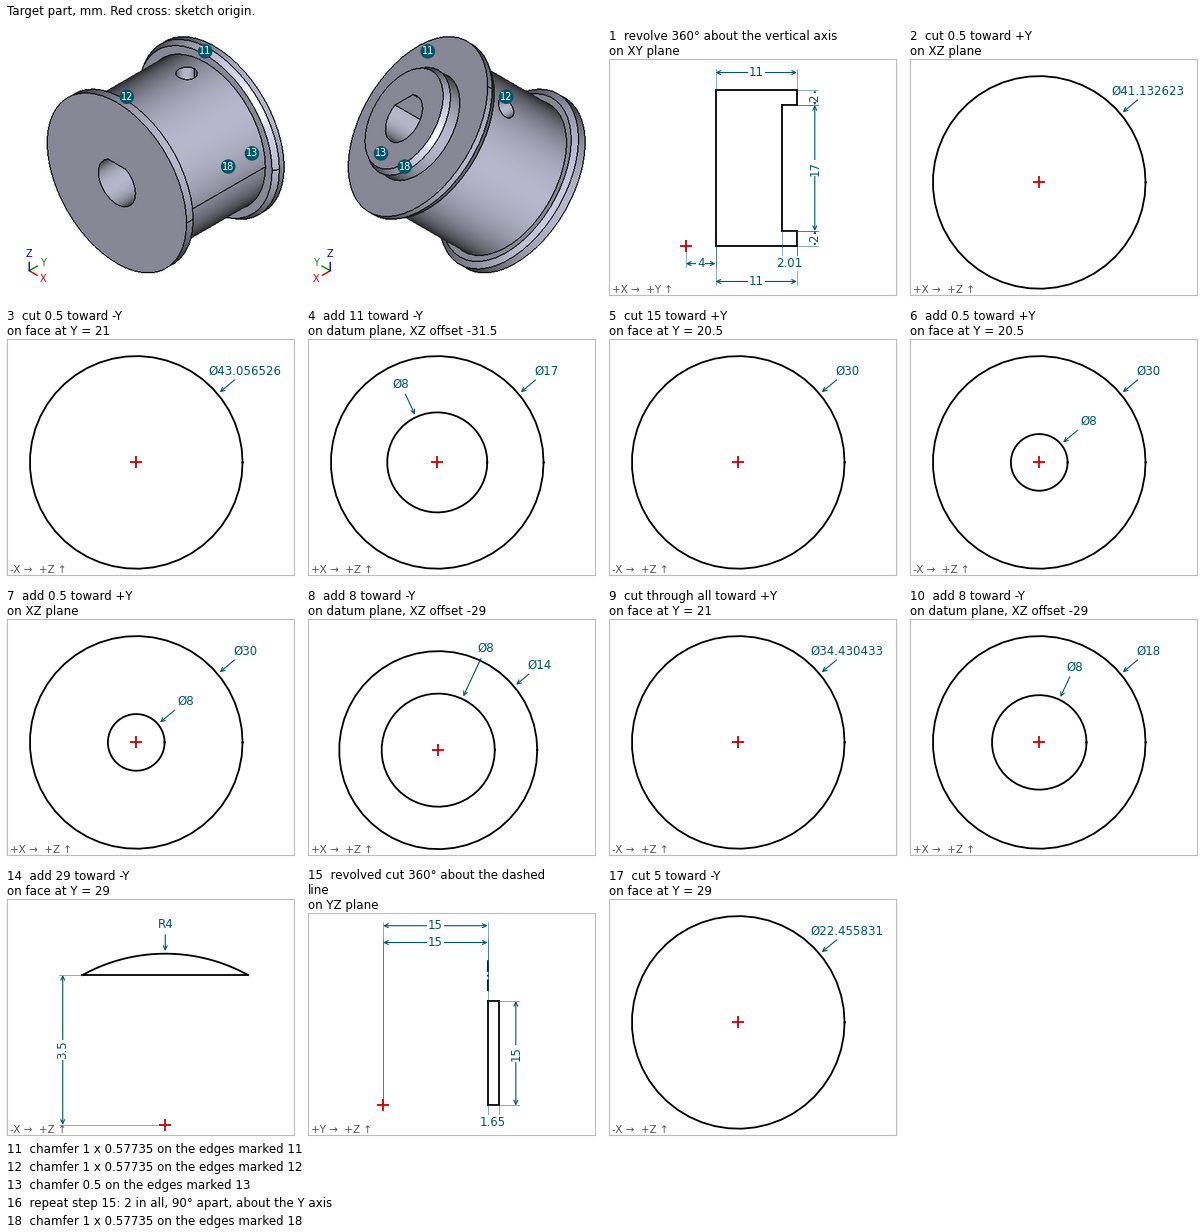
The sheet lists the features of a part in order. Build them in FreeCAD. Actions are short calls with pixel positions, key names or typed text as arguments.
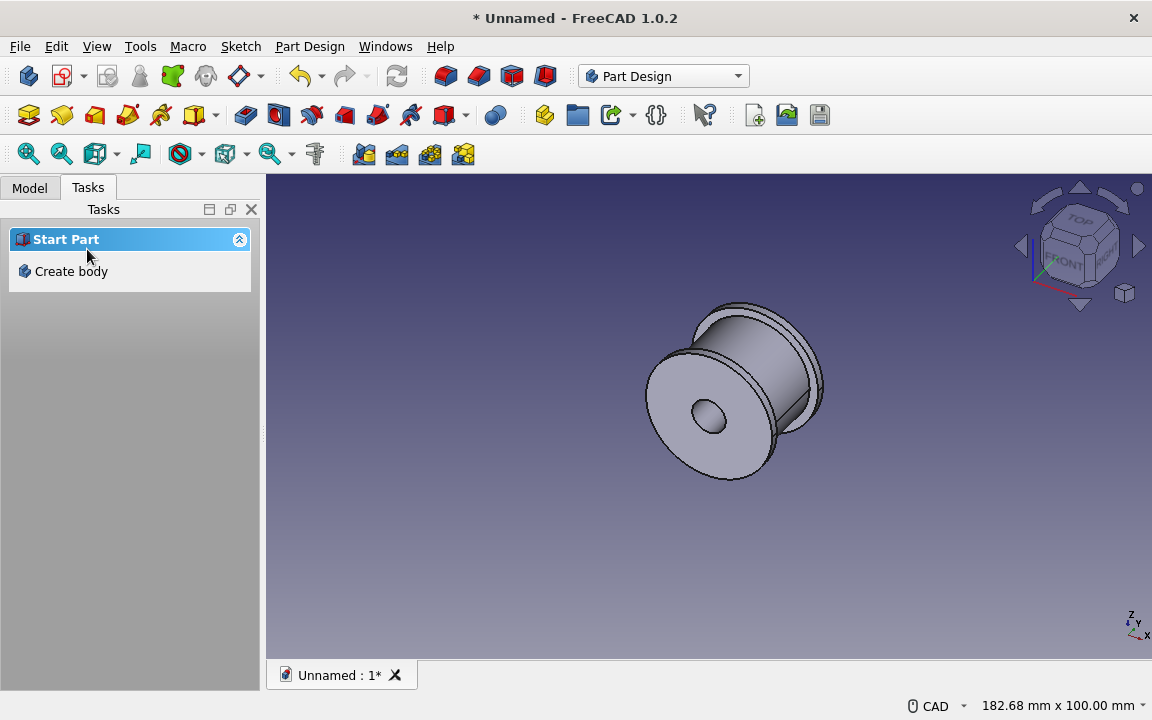
click(29, 154)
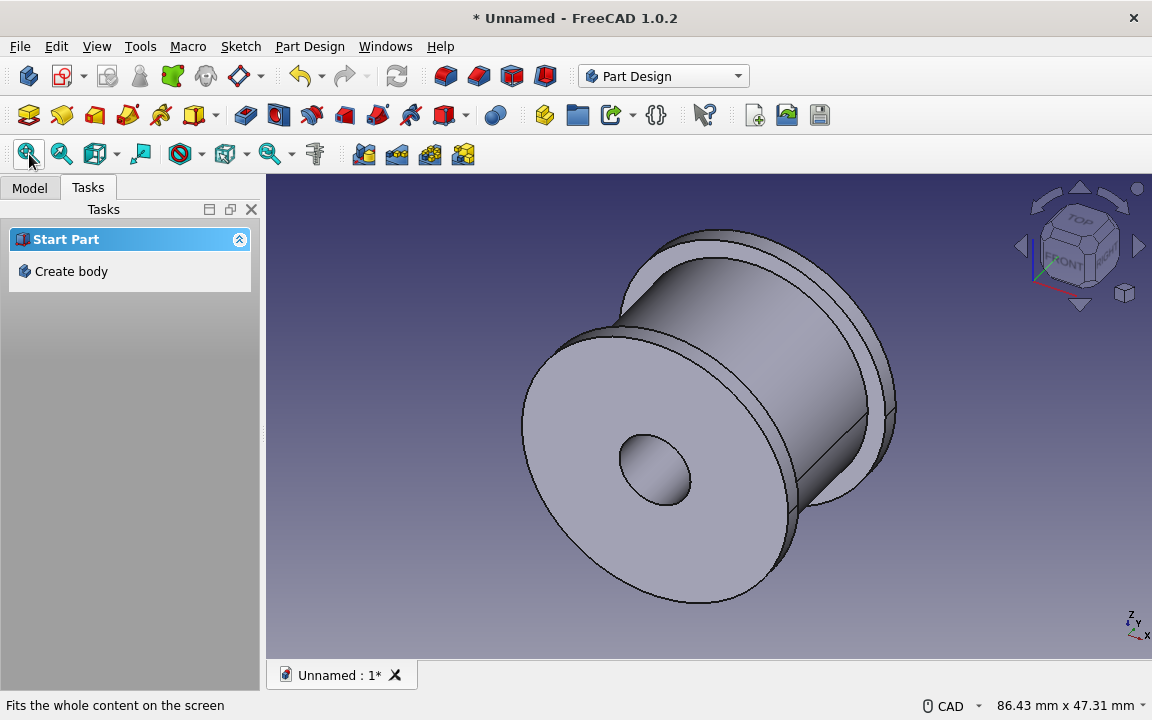
click(62, 76)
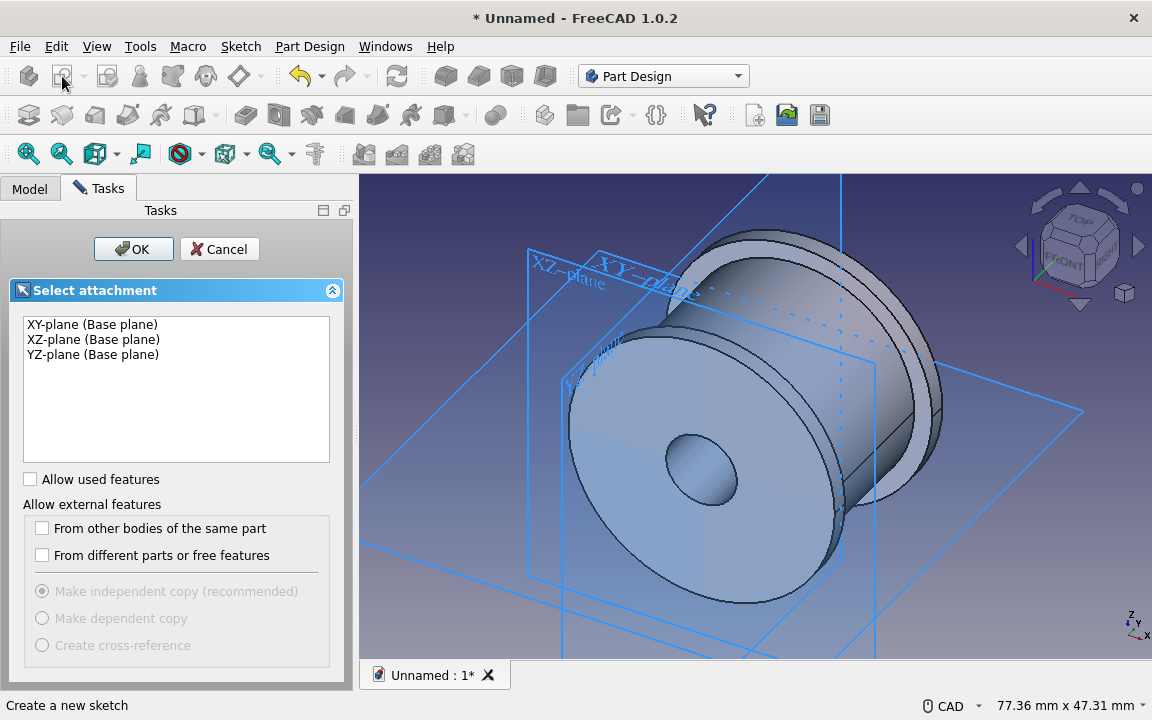
click(84, 340)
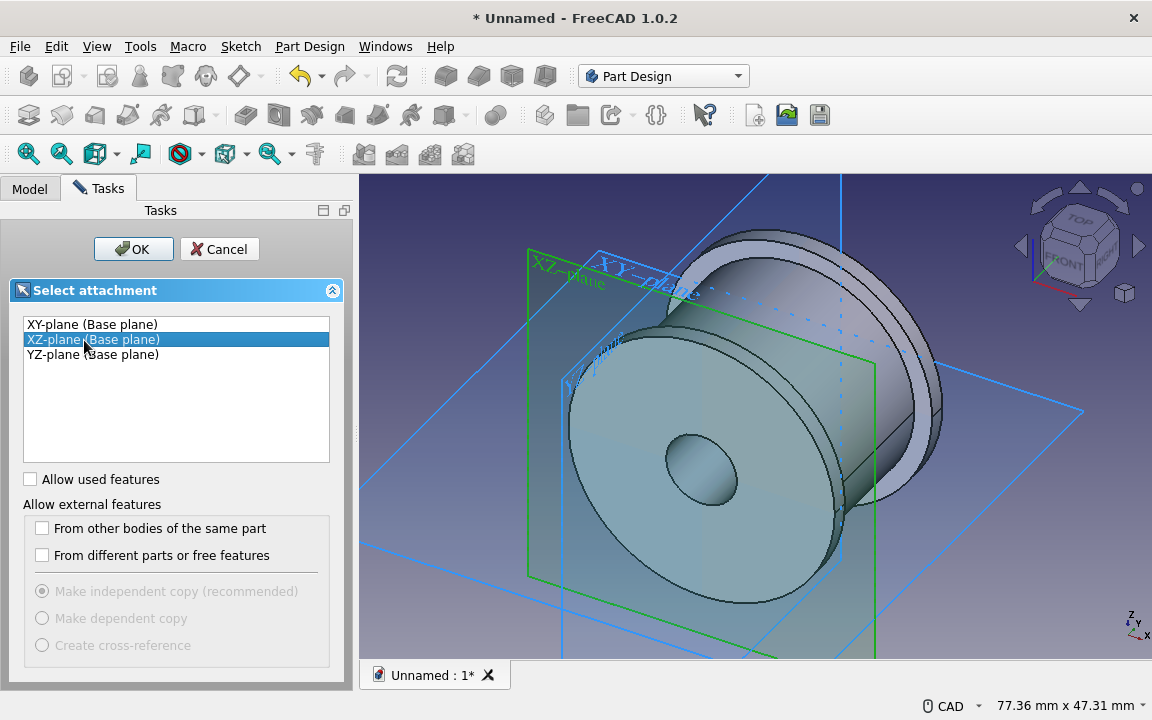
click(134, 249)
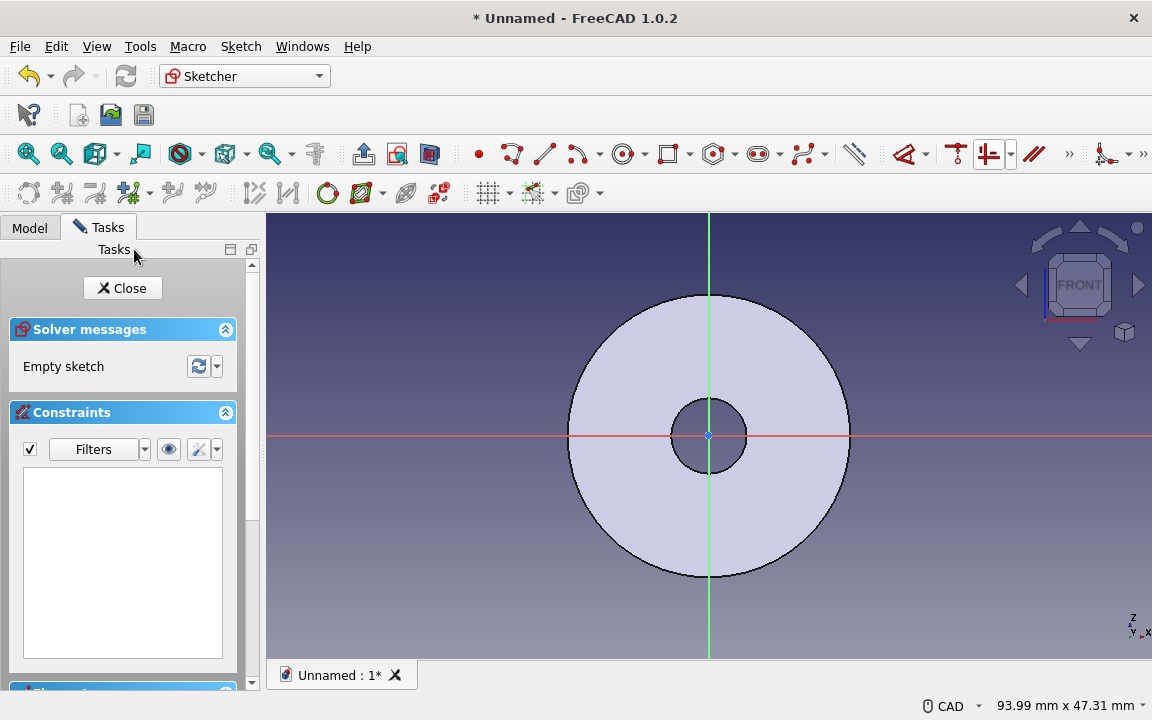
scroll(501, 436, down, 2)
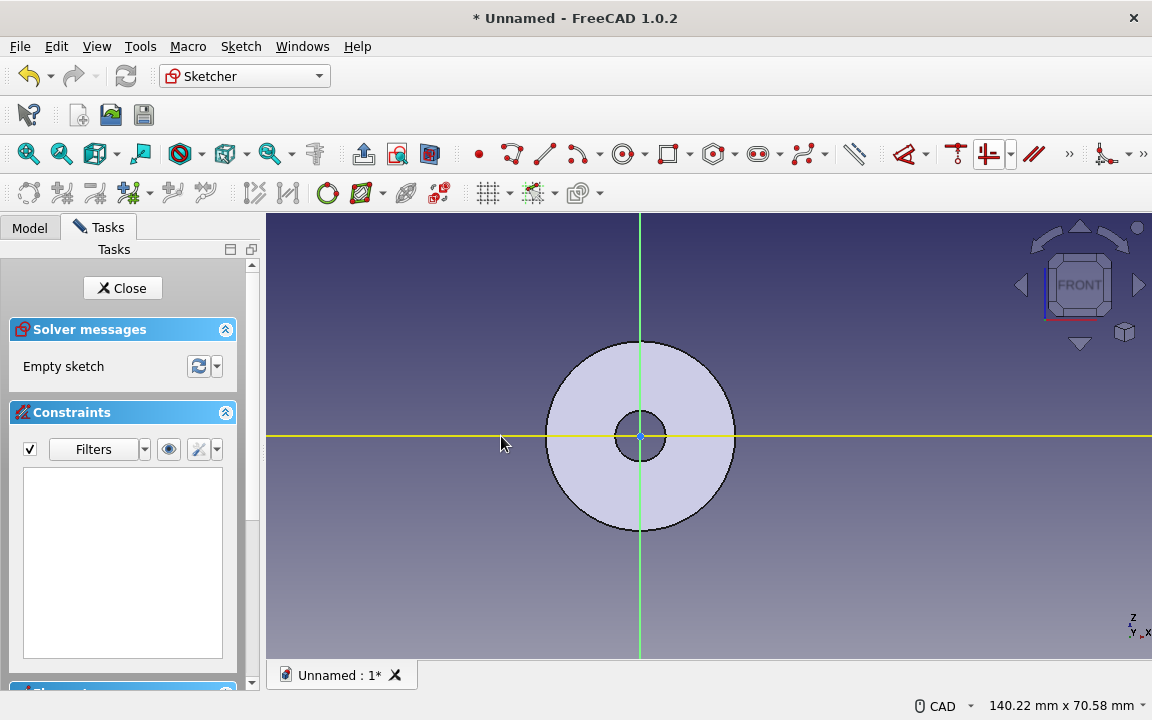
click(622, 154)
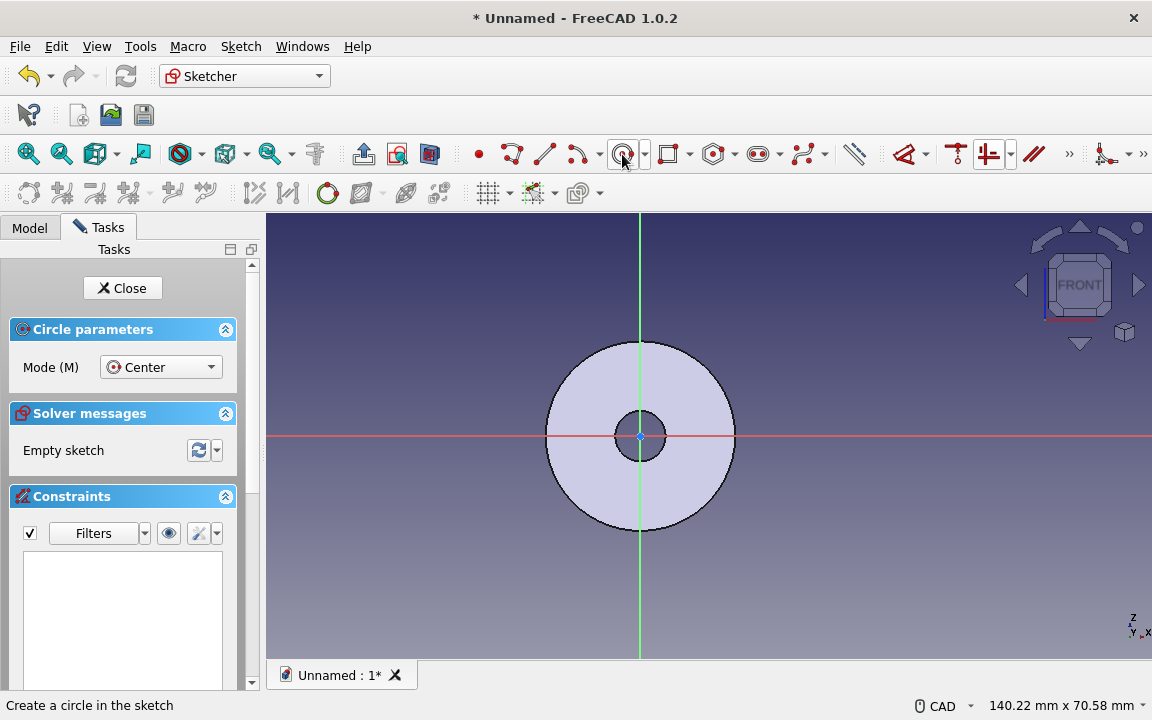
click(640, 436)
move(732, 344)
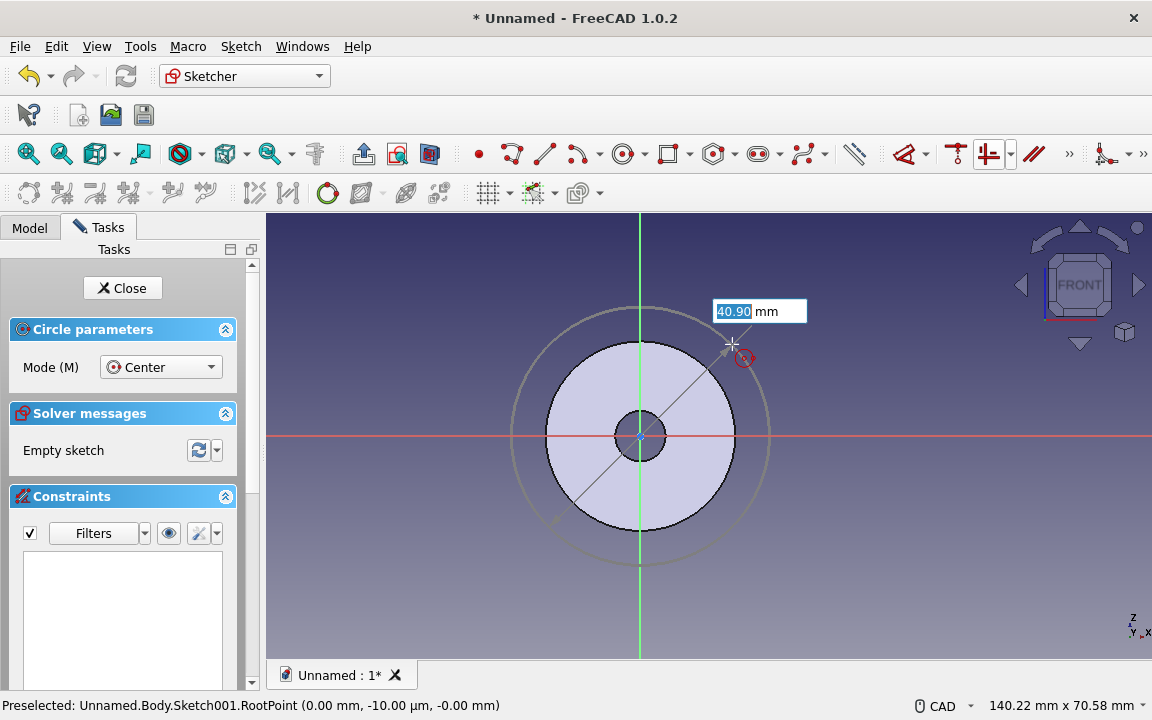
text(41.132623)
key(Return)
key(Escape)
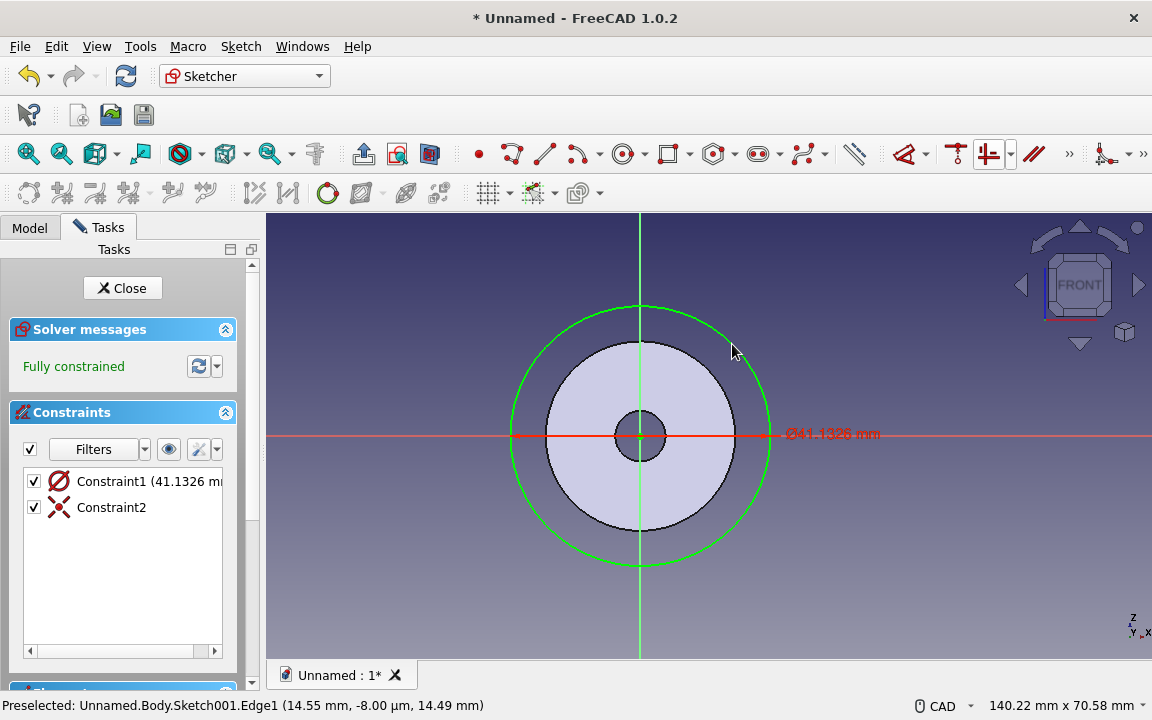
click(123, 288)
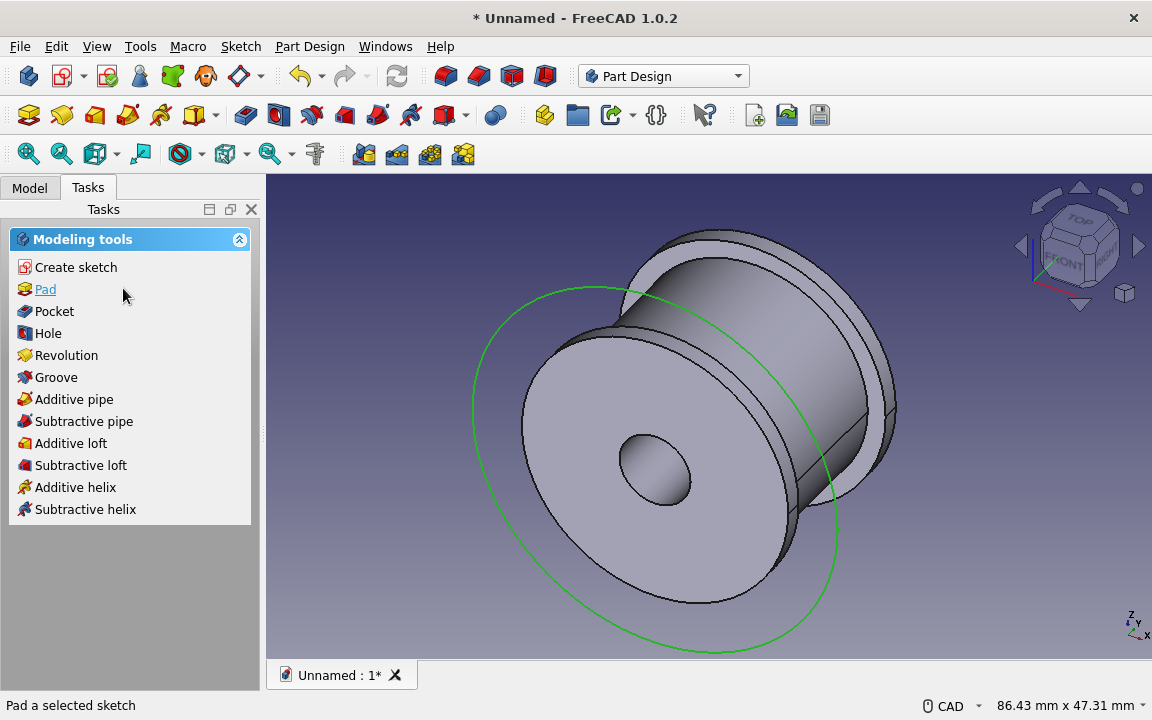
click(246, 116)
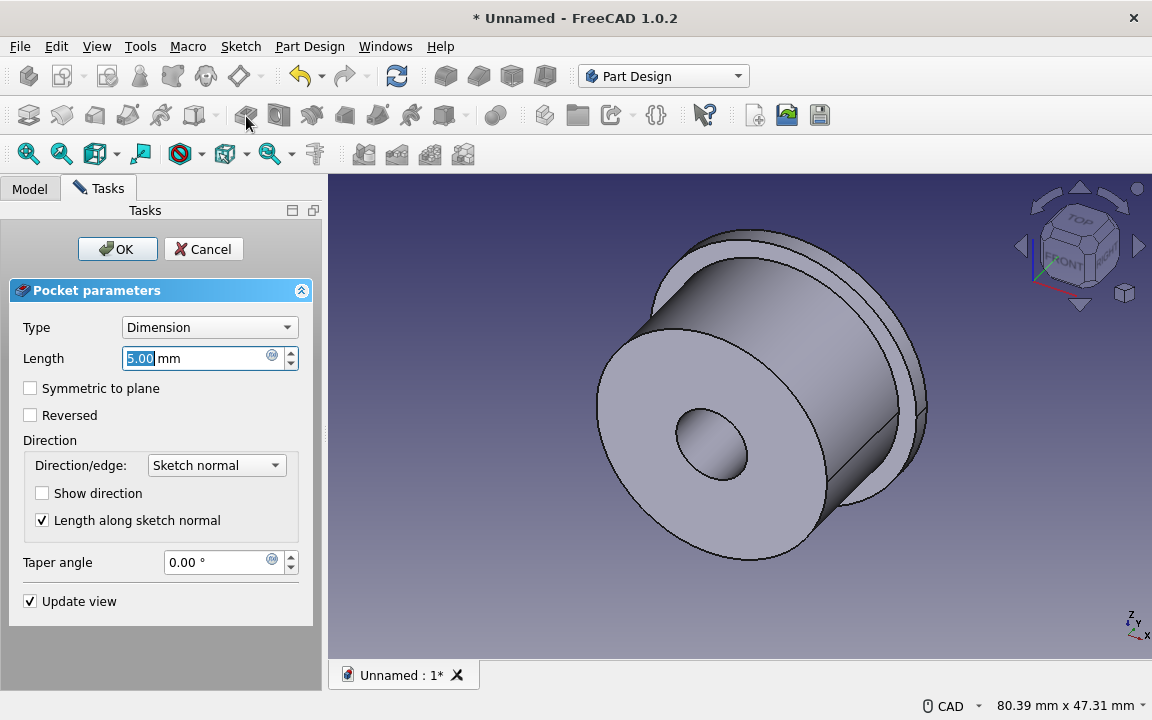
text(0.5)
key(Tab)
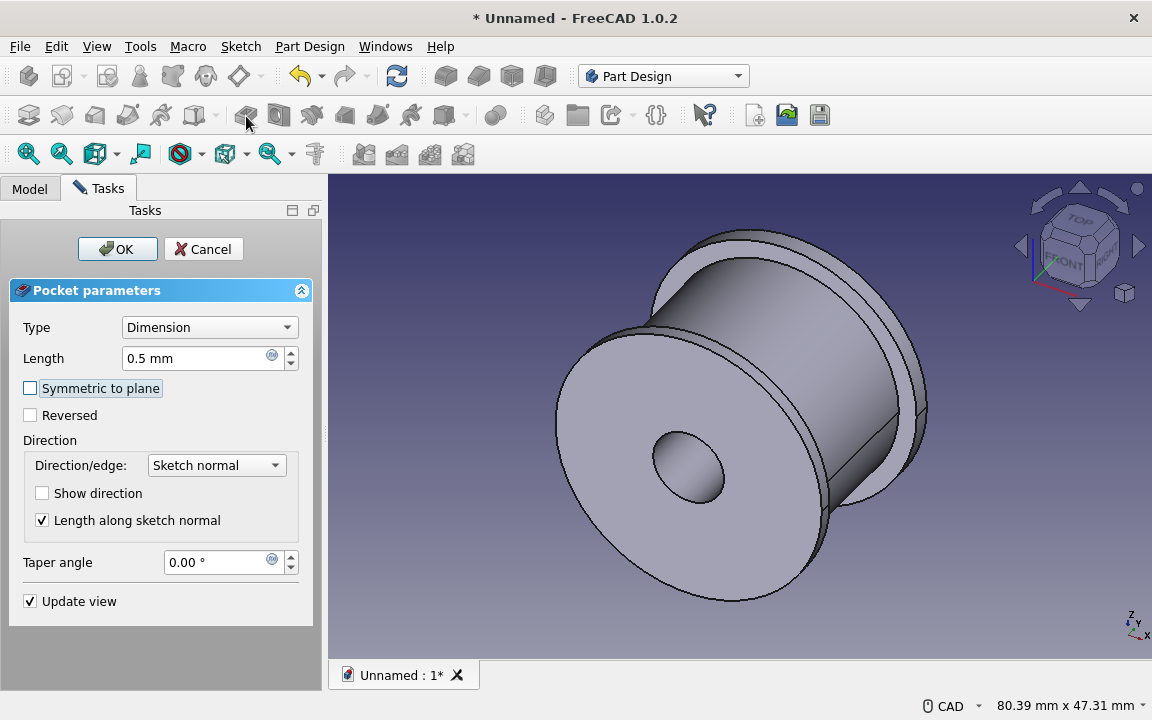
click(118, 249)